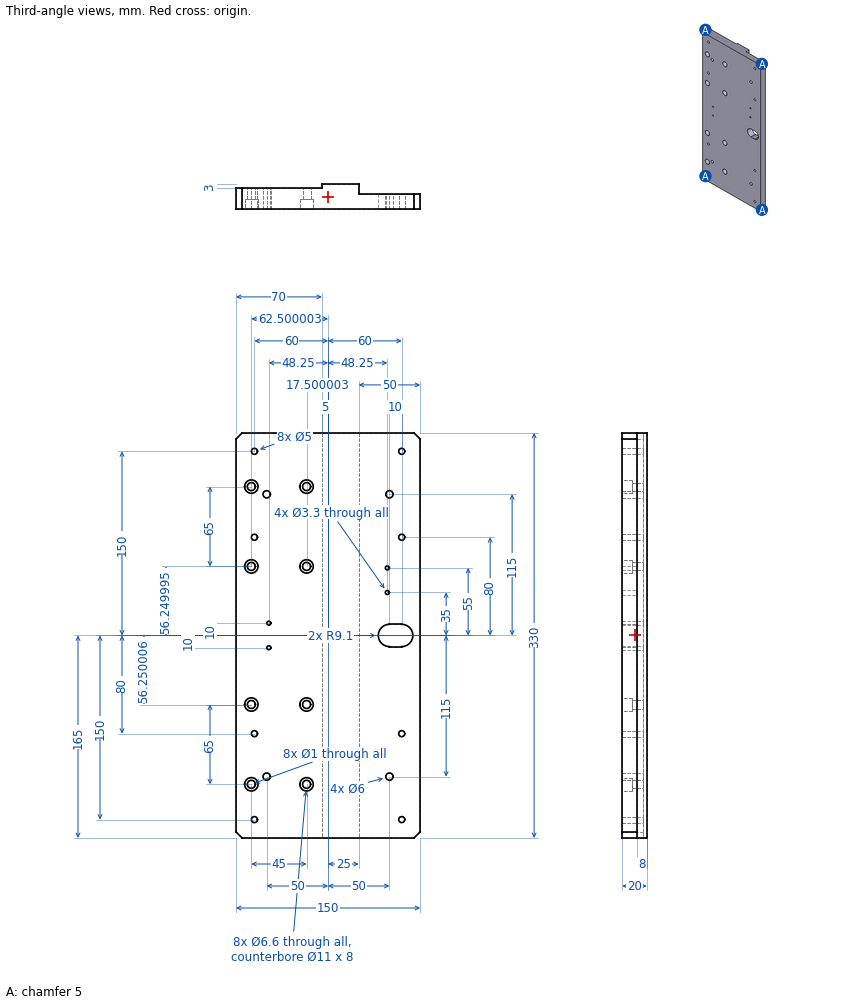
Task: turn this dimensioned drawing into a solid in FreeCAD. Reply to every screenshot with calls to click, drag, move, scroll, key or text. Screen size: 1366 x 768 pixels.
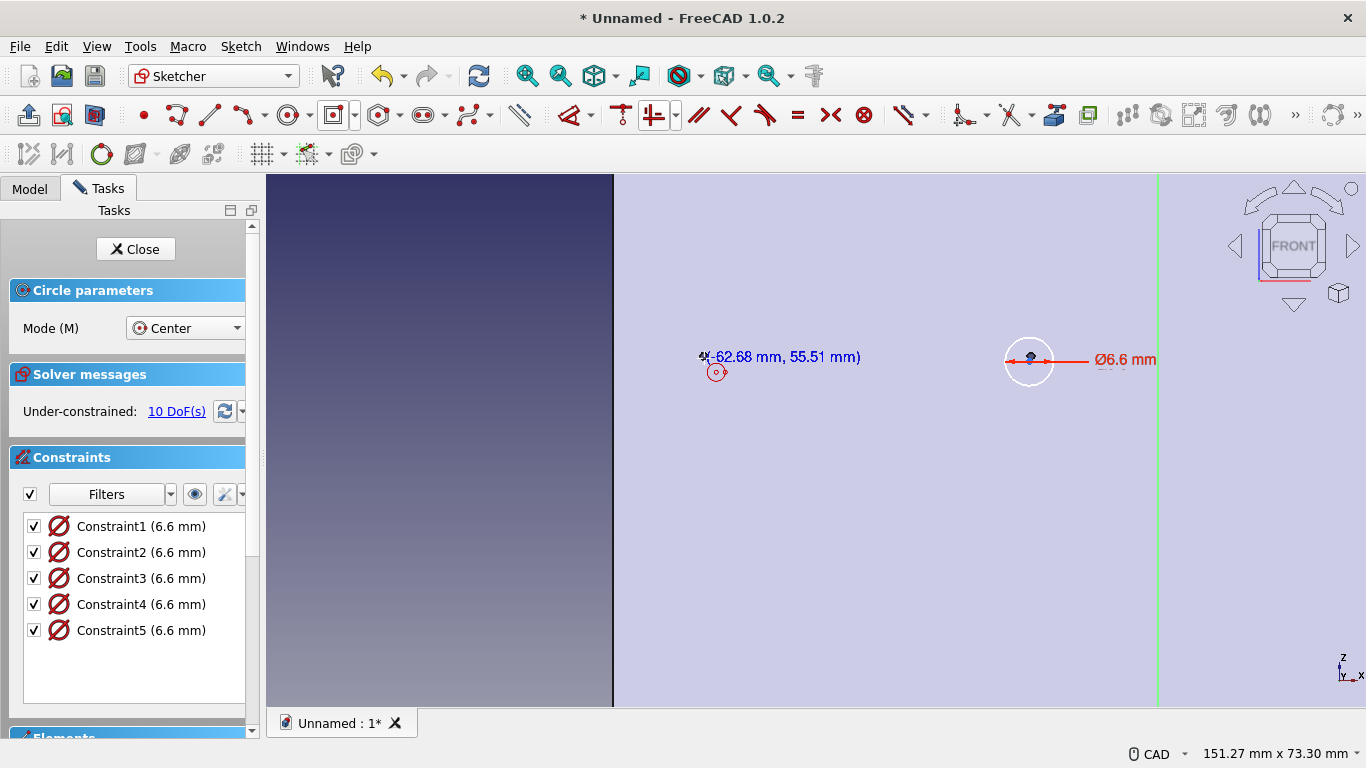
scroll(704, 358, down, 8)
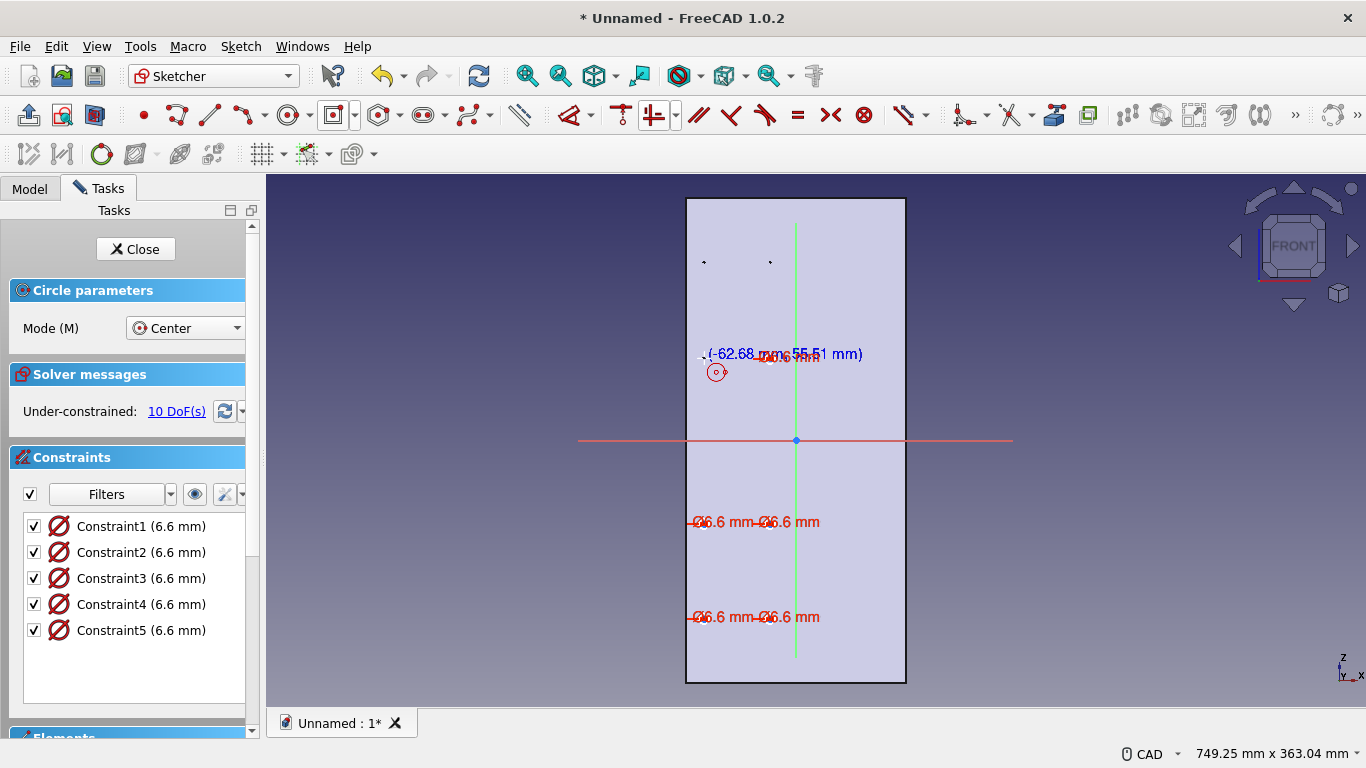
click(704, 358)
move(708, 354)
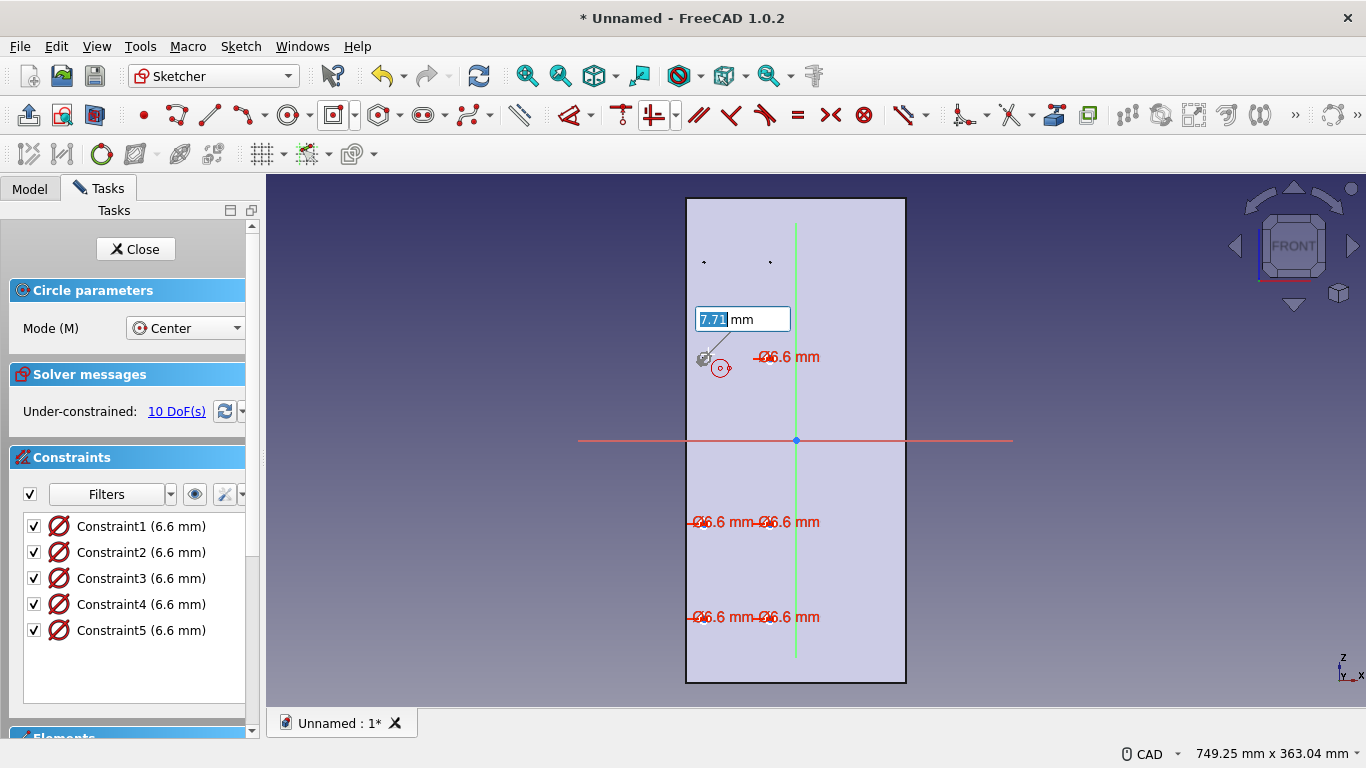
text(6.6)
key(Return)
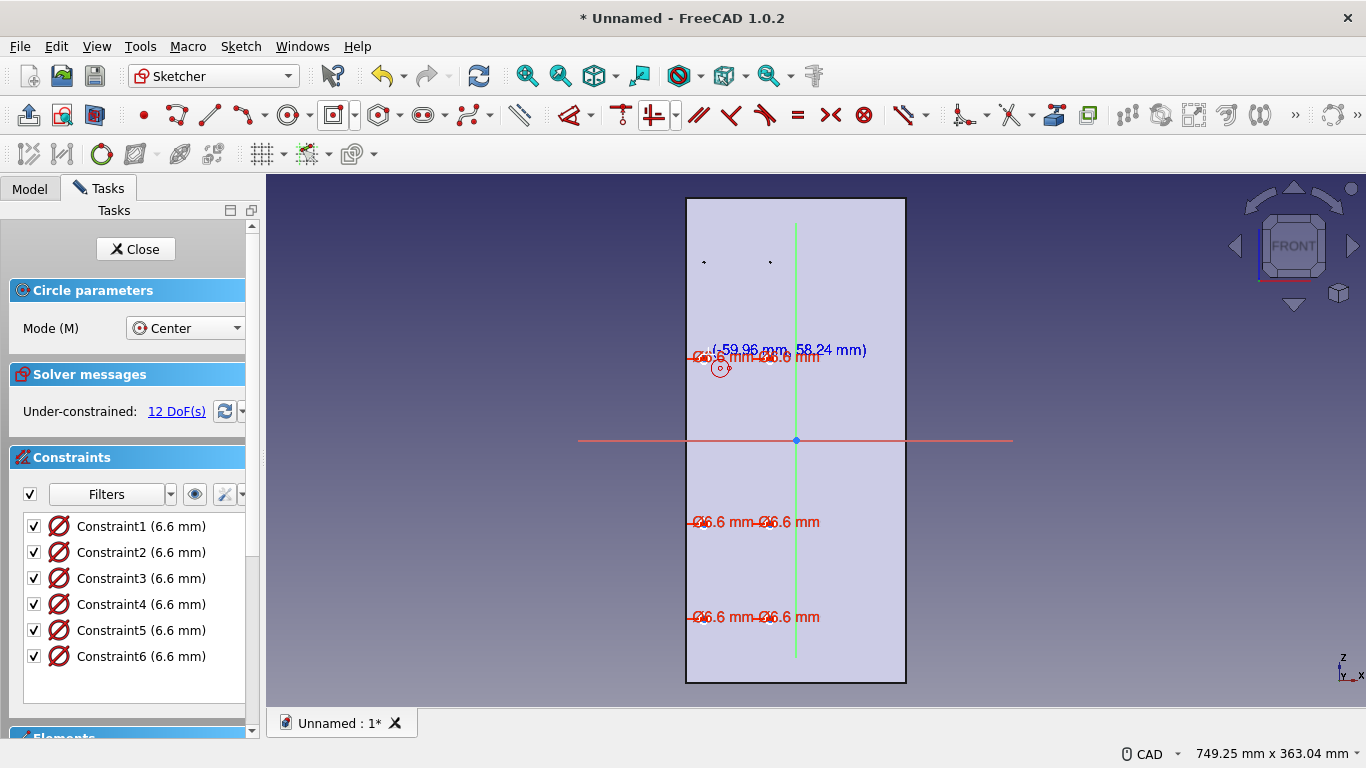
scroll(770, 262, up, 8)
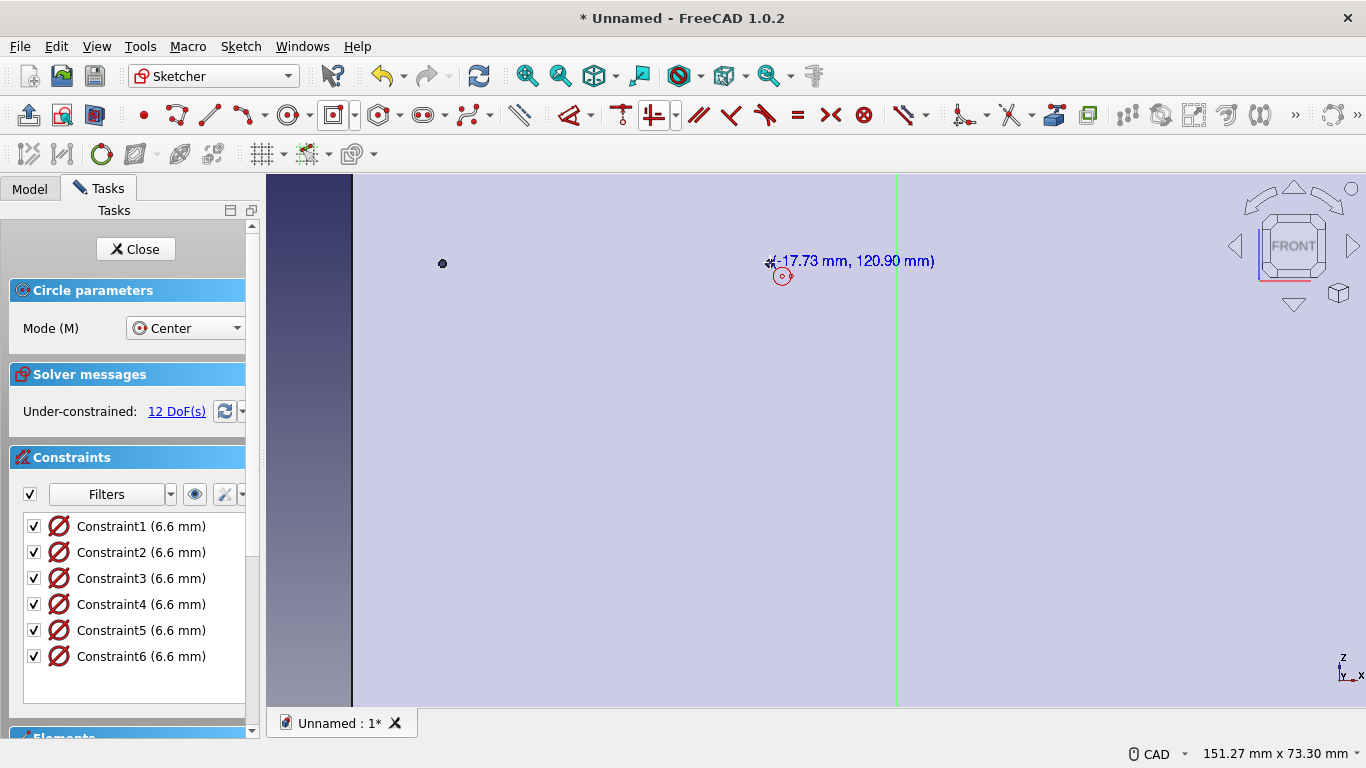
scroll(770, 262, down, 8)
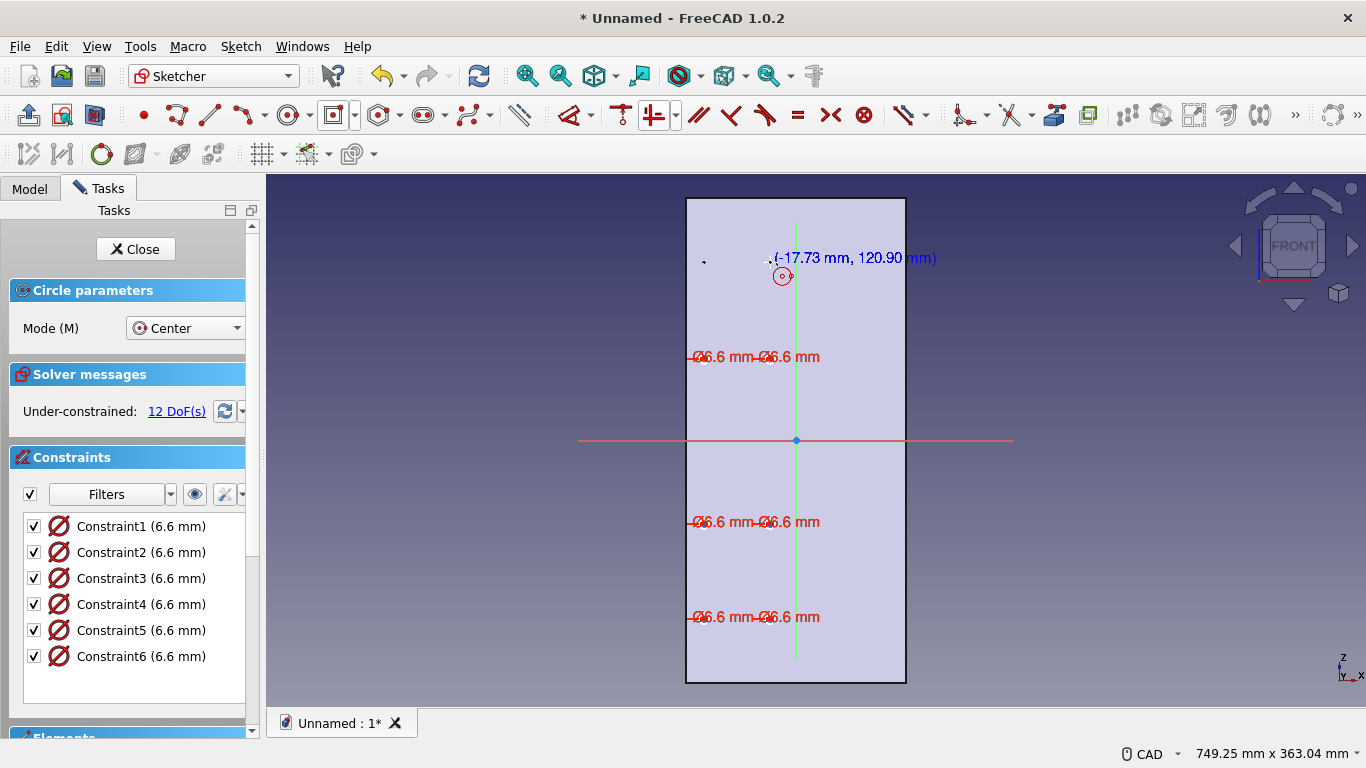
click(770, 262)
move(774, 259)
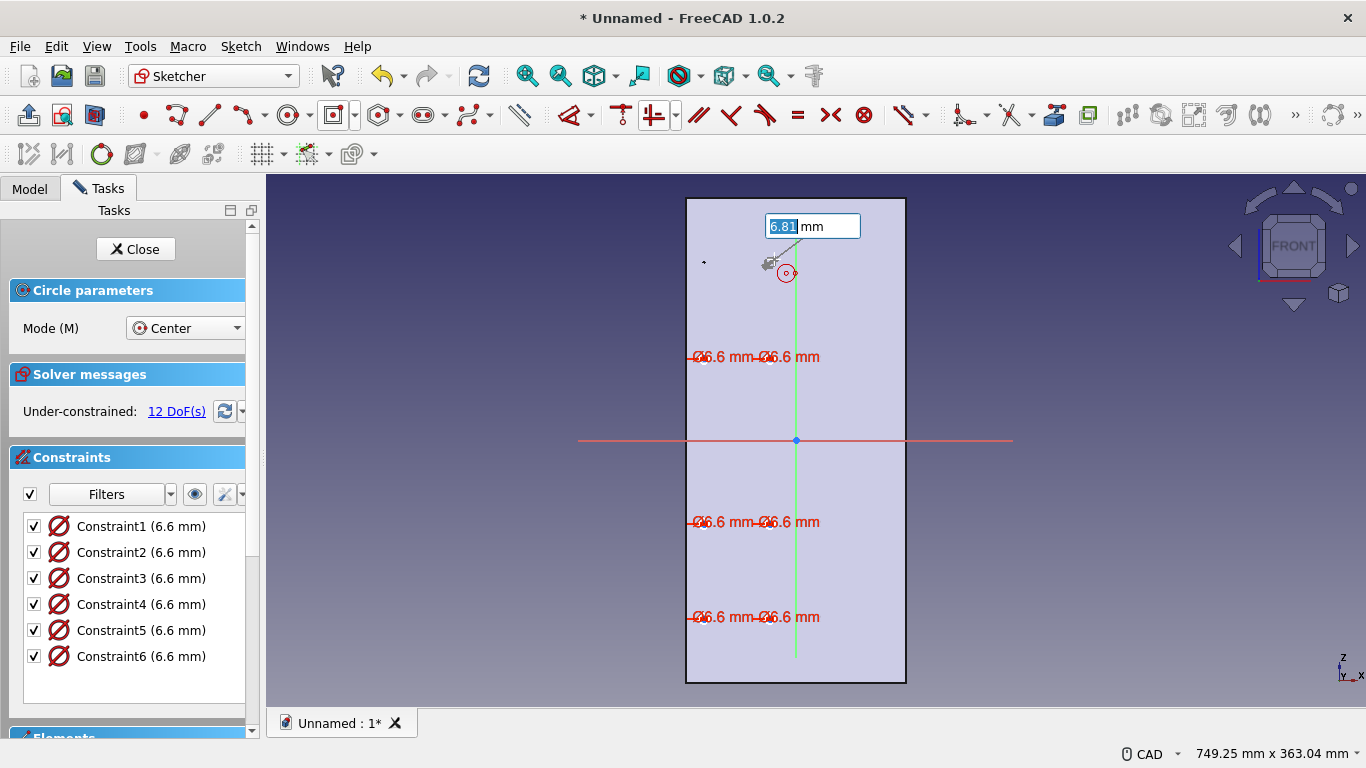
text(6.6)
key(Return)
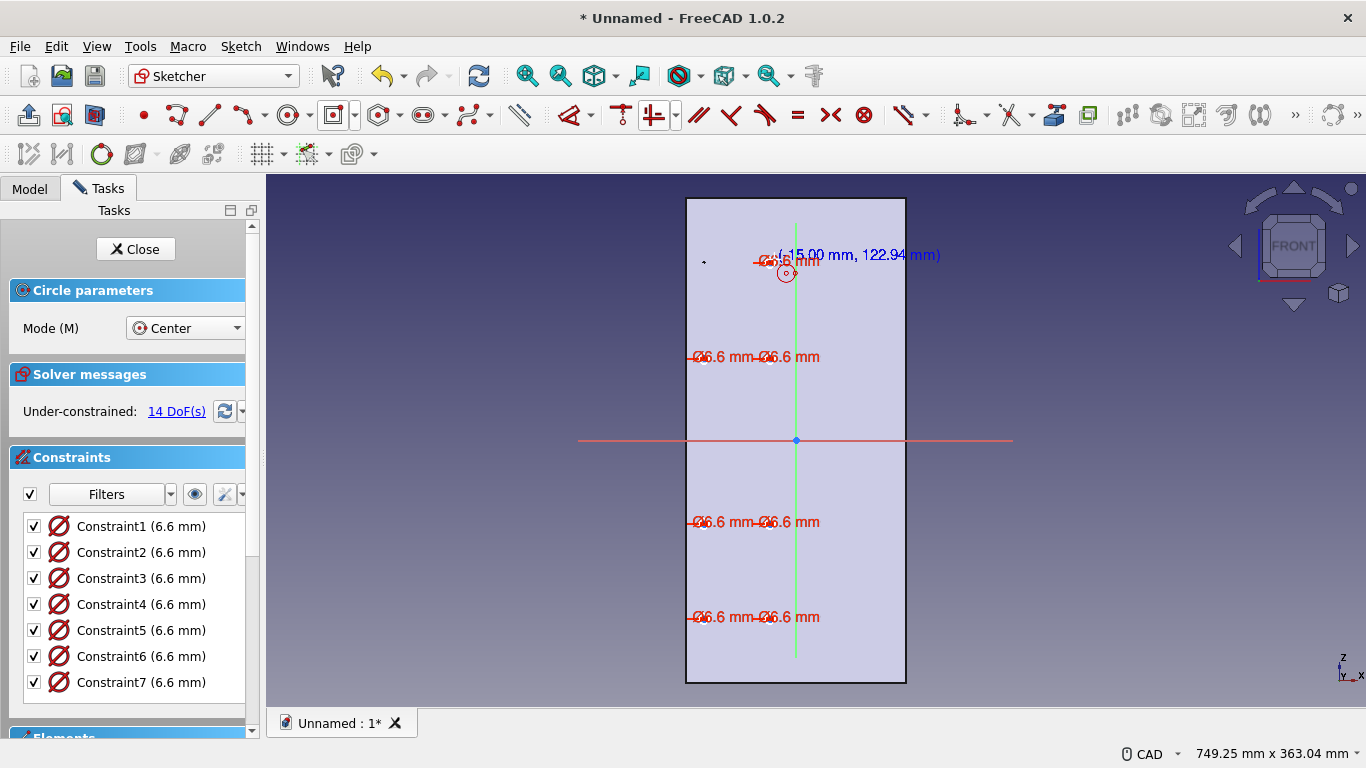
scroll(704, 262, up, 8)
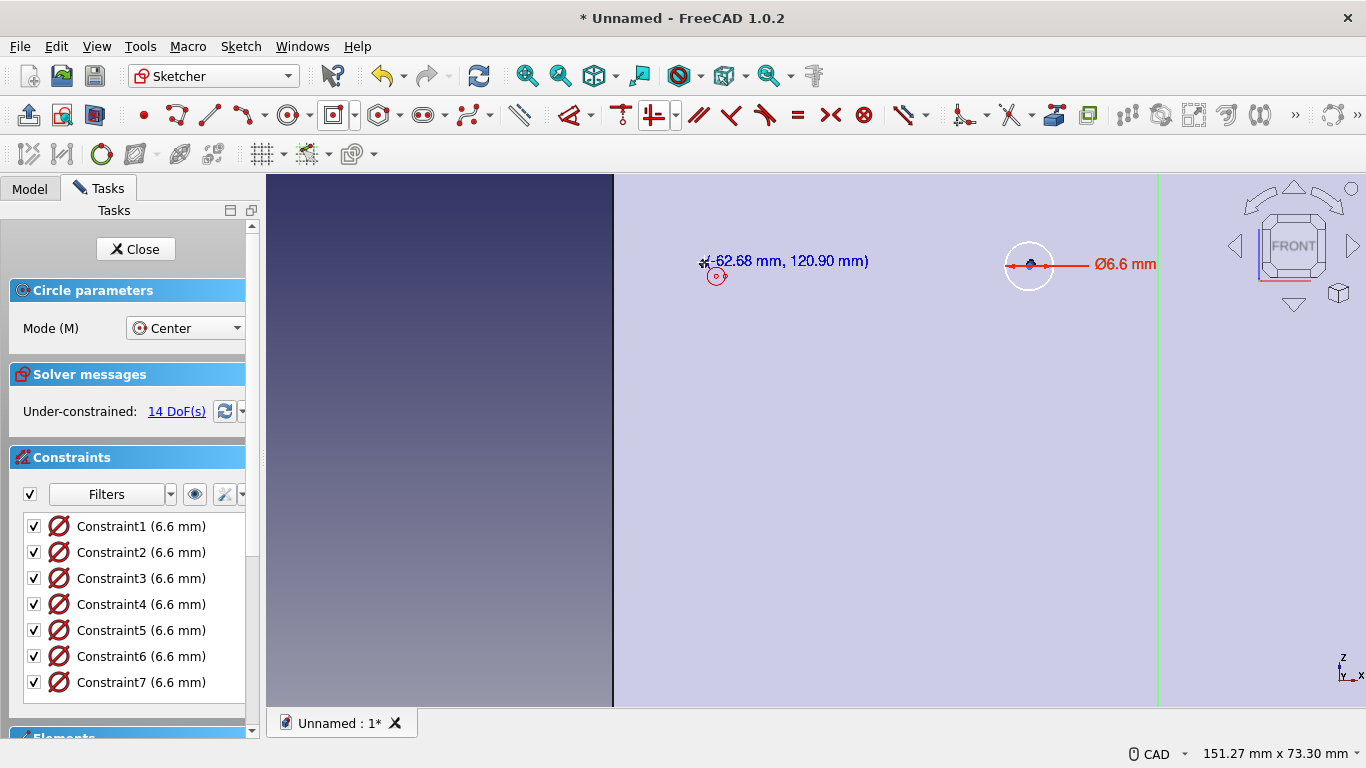
scroll(704, 262, down, 8)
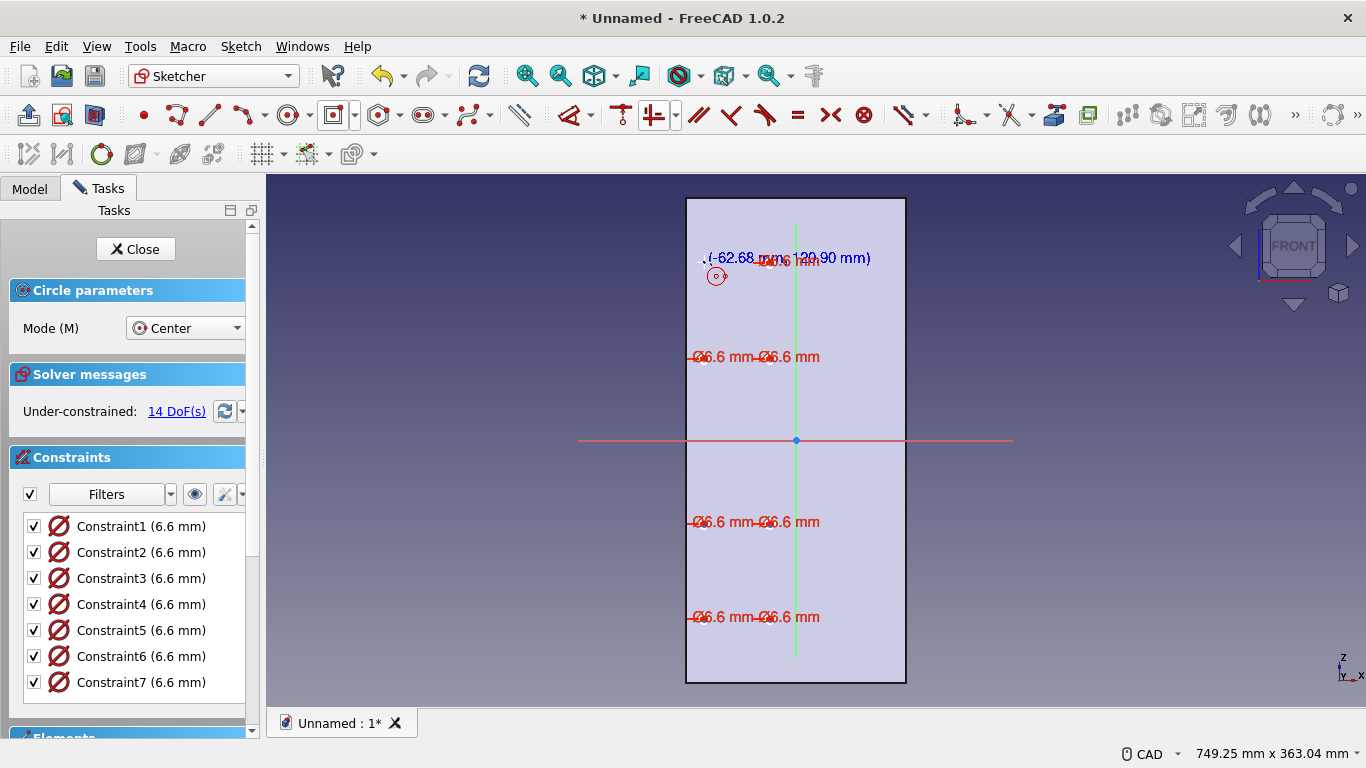
click(704, 262)
move(708, 259)